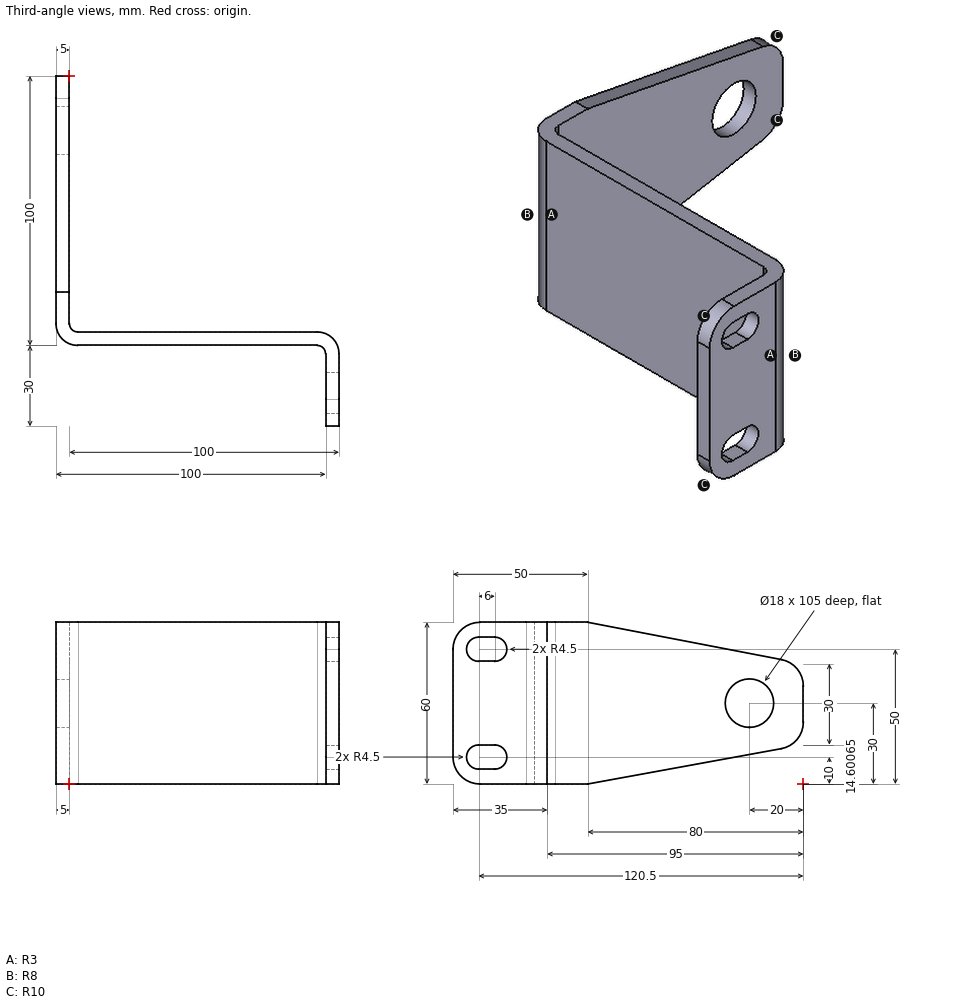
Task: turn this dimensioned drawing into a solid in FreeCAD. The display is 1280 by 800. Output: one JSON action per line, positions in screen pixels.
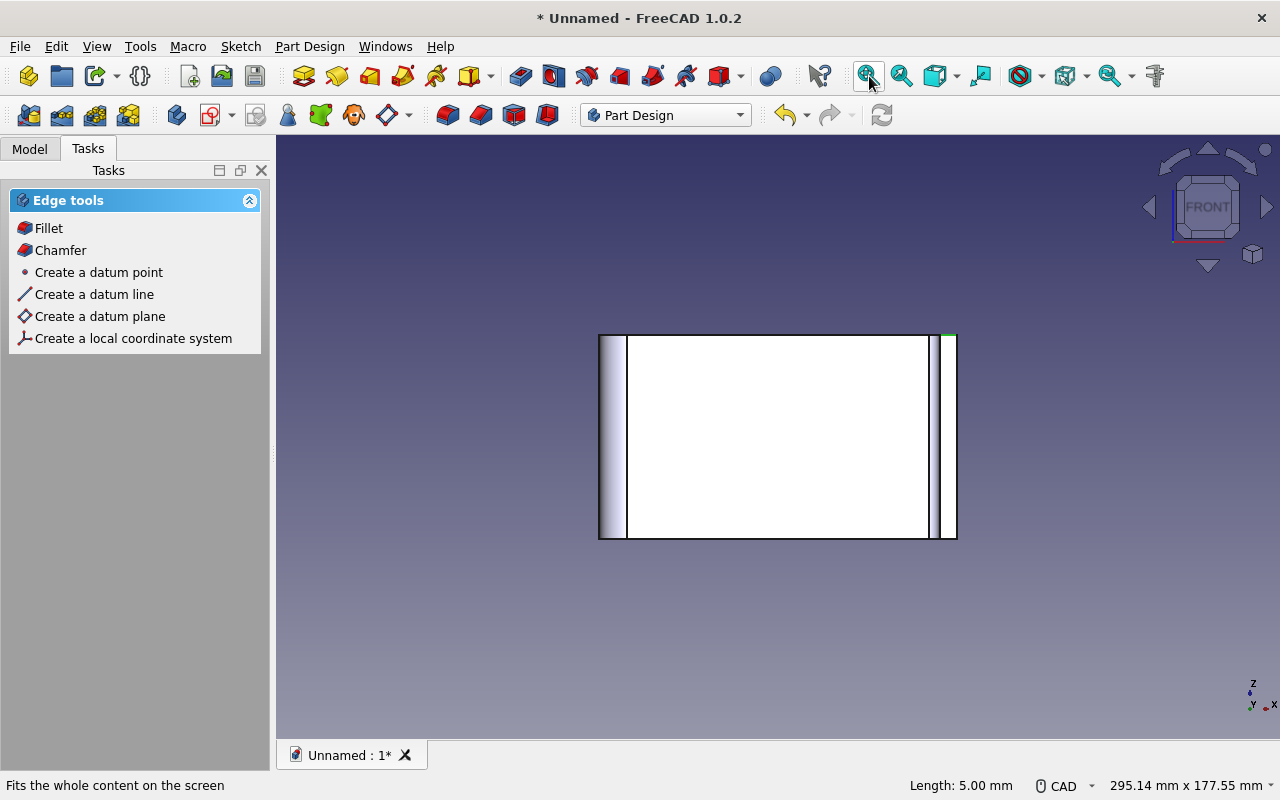
{"action": "left_click", "coordinate": [869, 76]}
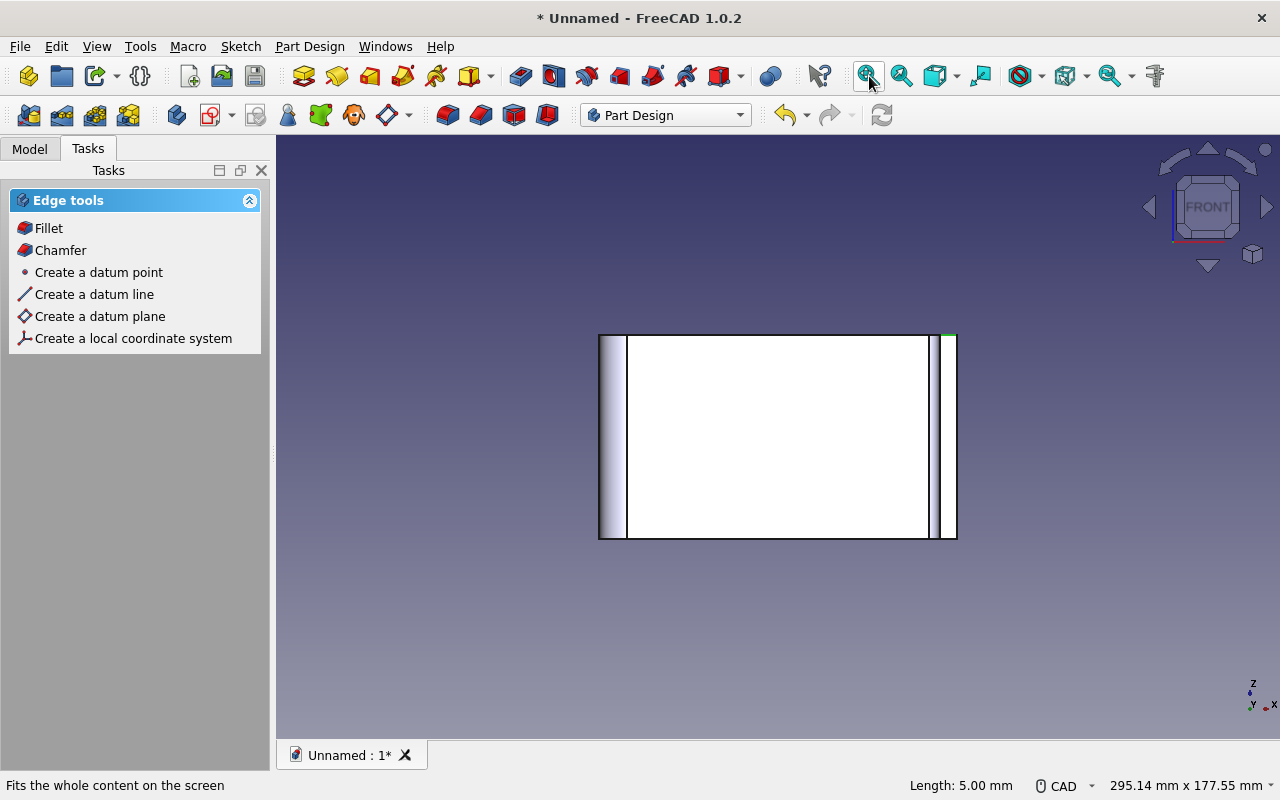
{"action": "left_click", "coordinate": [948, 538], "text": "ctrl"}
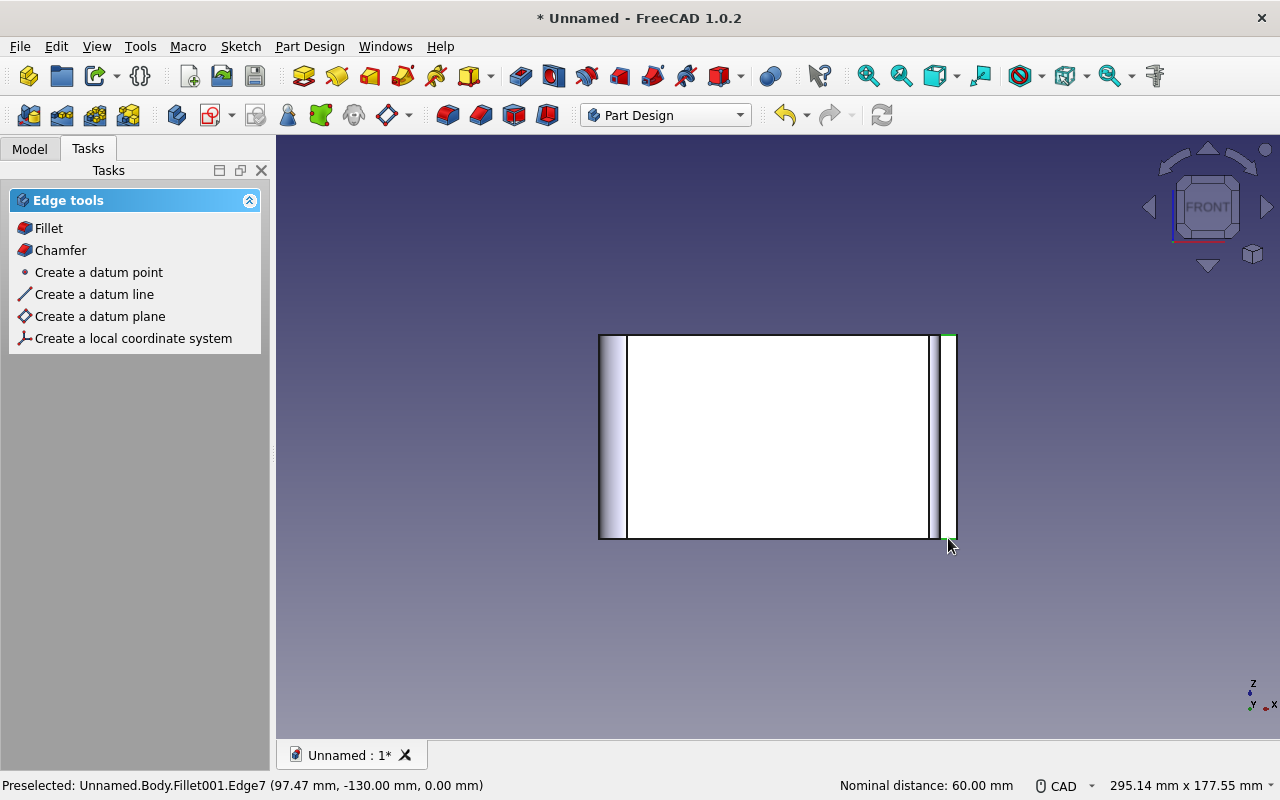
{"action": "scroll", "coordinate": [608, 386], "scroll_direction": "up", "scroll_amount": 5}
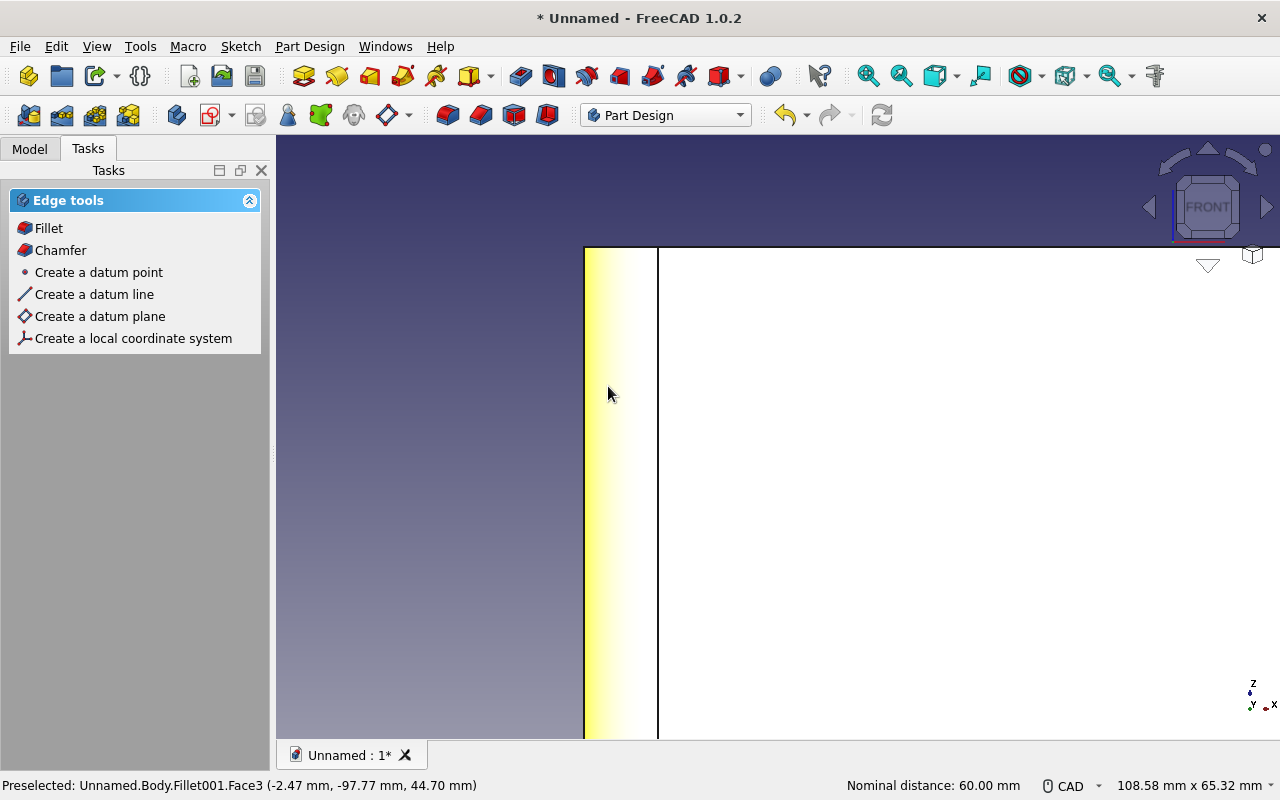
{"action": "left_click", "coordinate": [869, 76]}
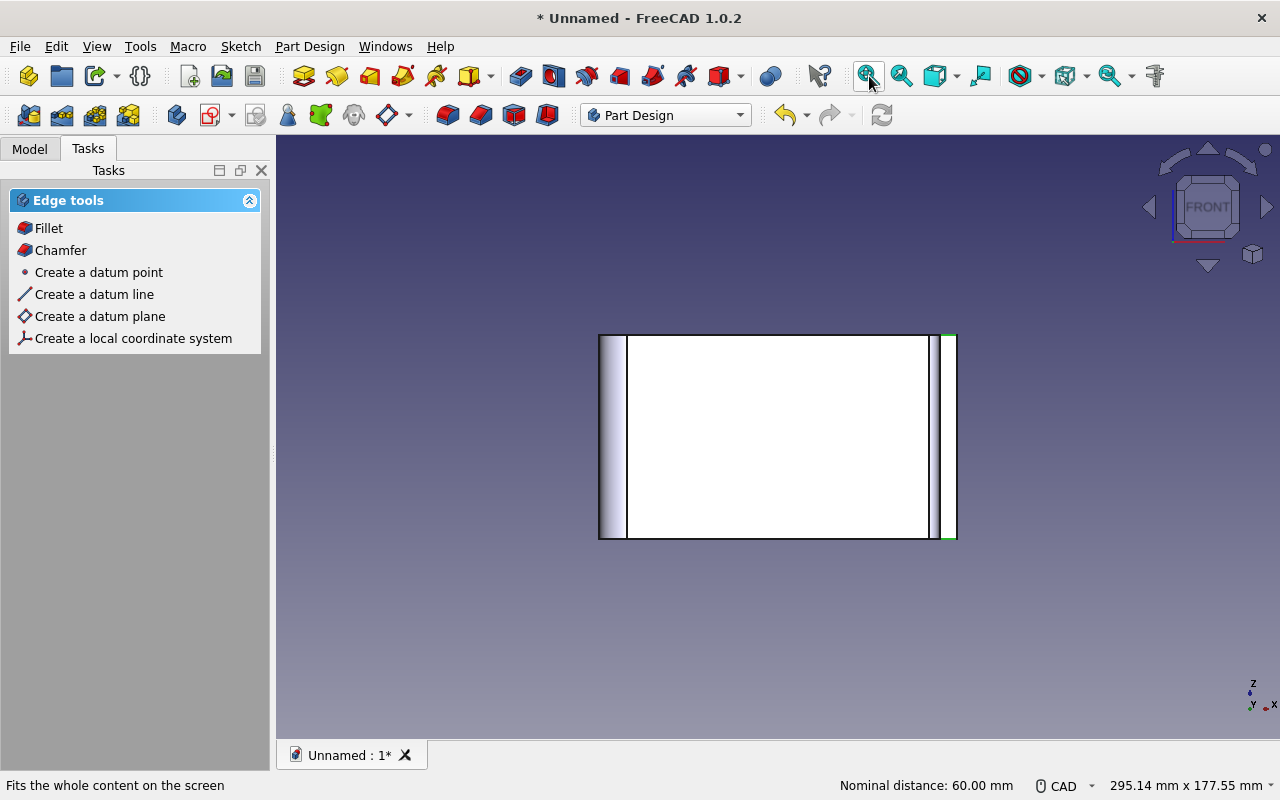
{"action": "key", "text": "3"}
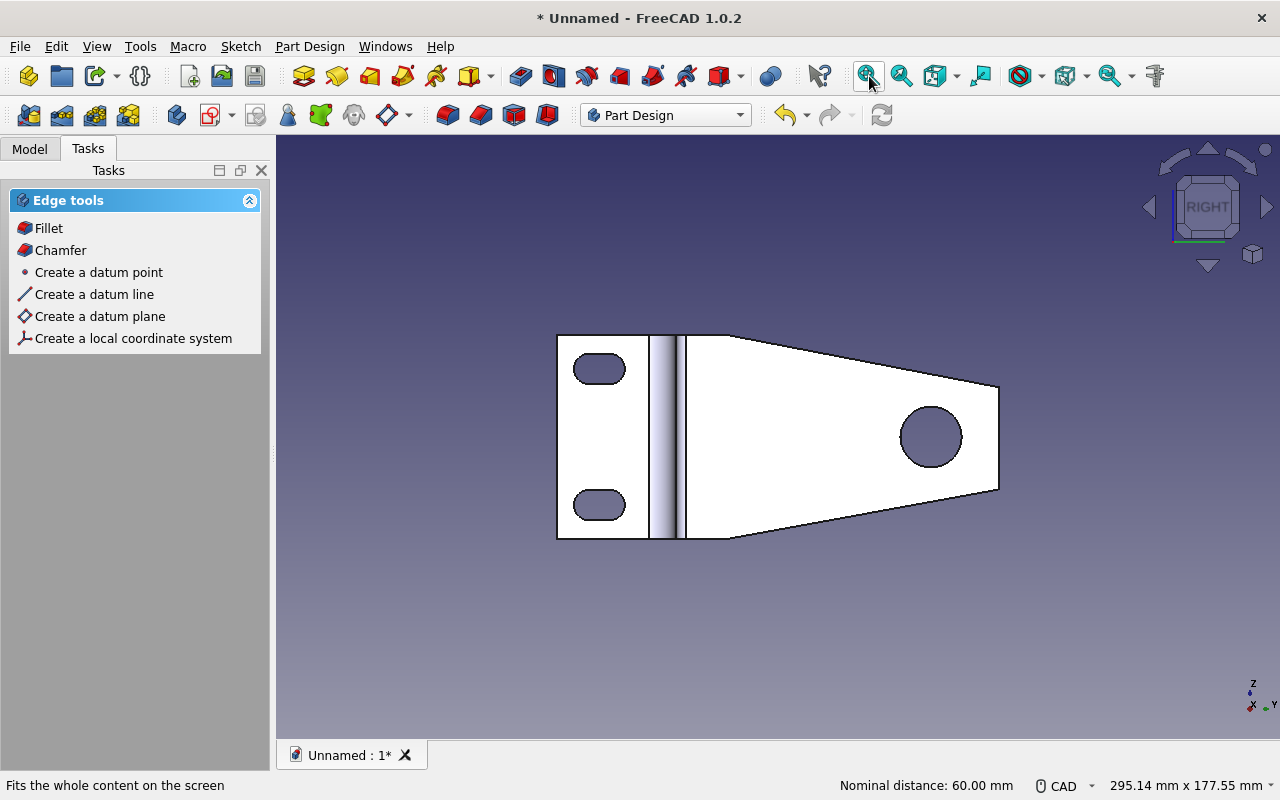
{"action": "left_click", "coordinate": [869, 76]}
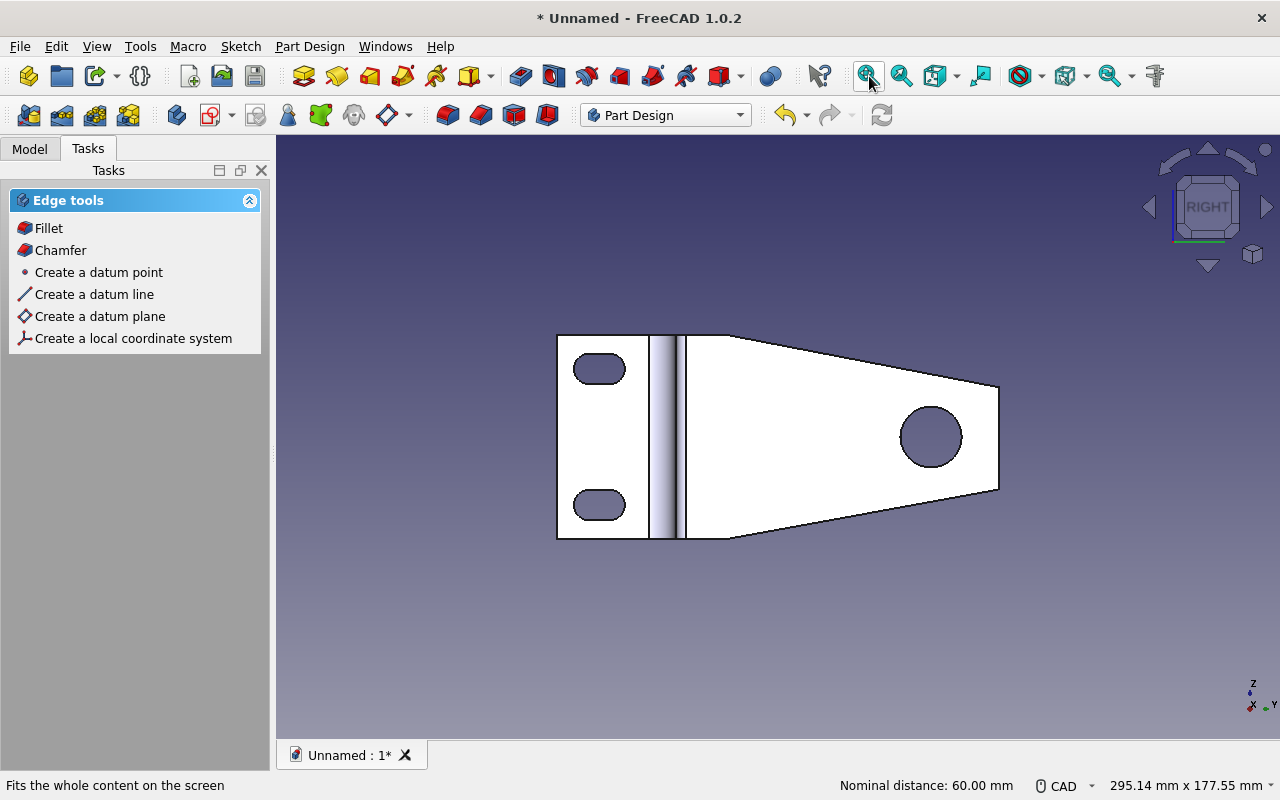
{"action": "scroll", "coordinate": [999, 386], "scroll_direction": "up", "scroll_amount": 5}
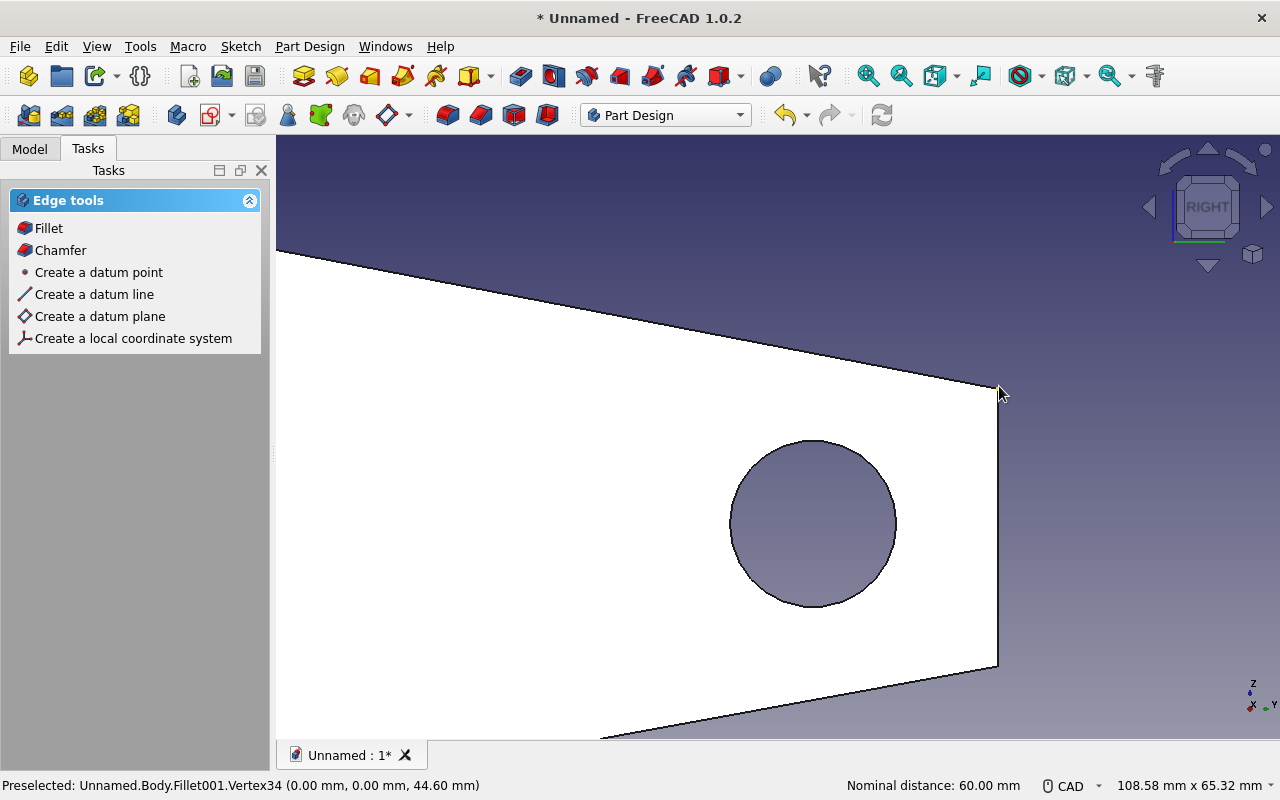
{"action": "left_click", "coordinate": [869, 76]}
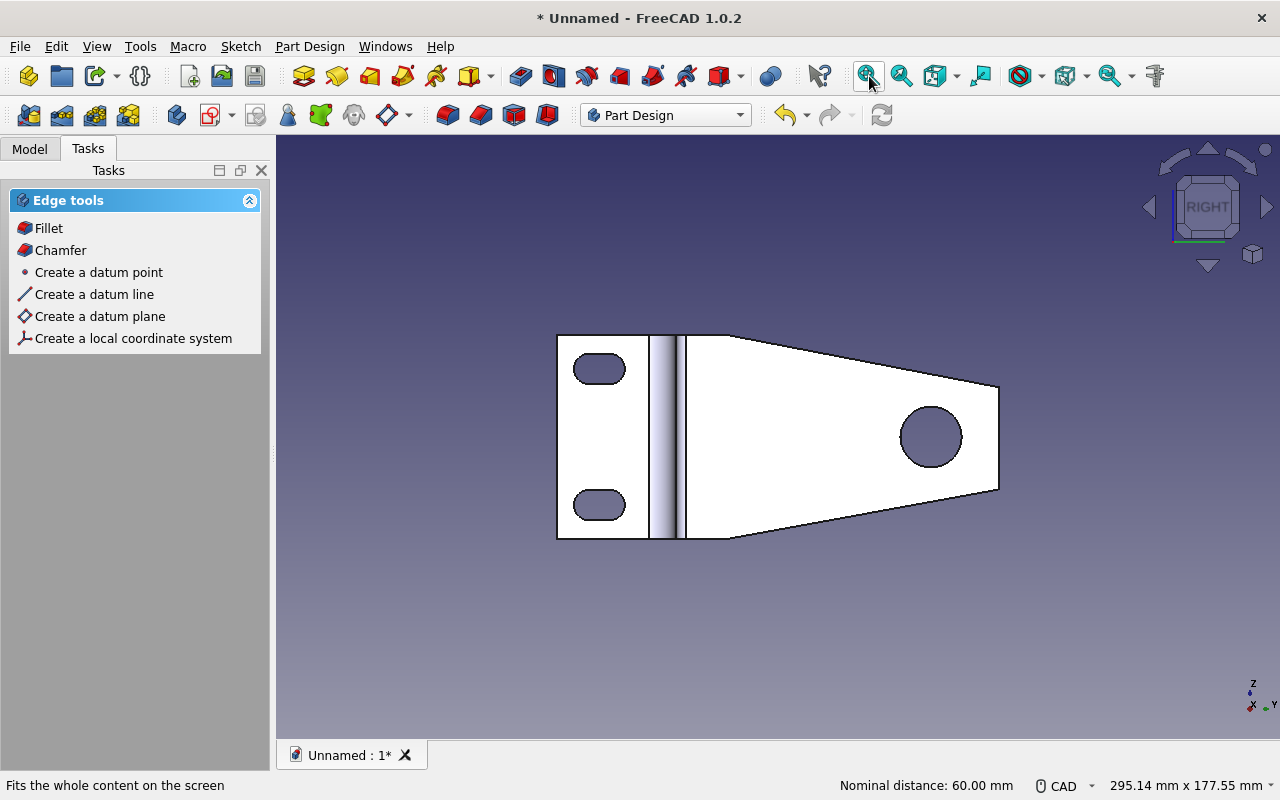
{"action": "key", "text": "5"}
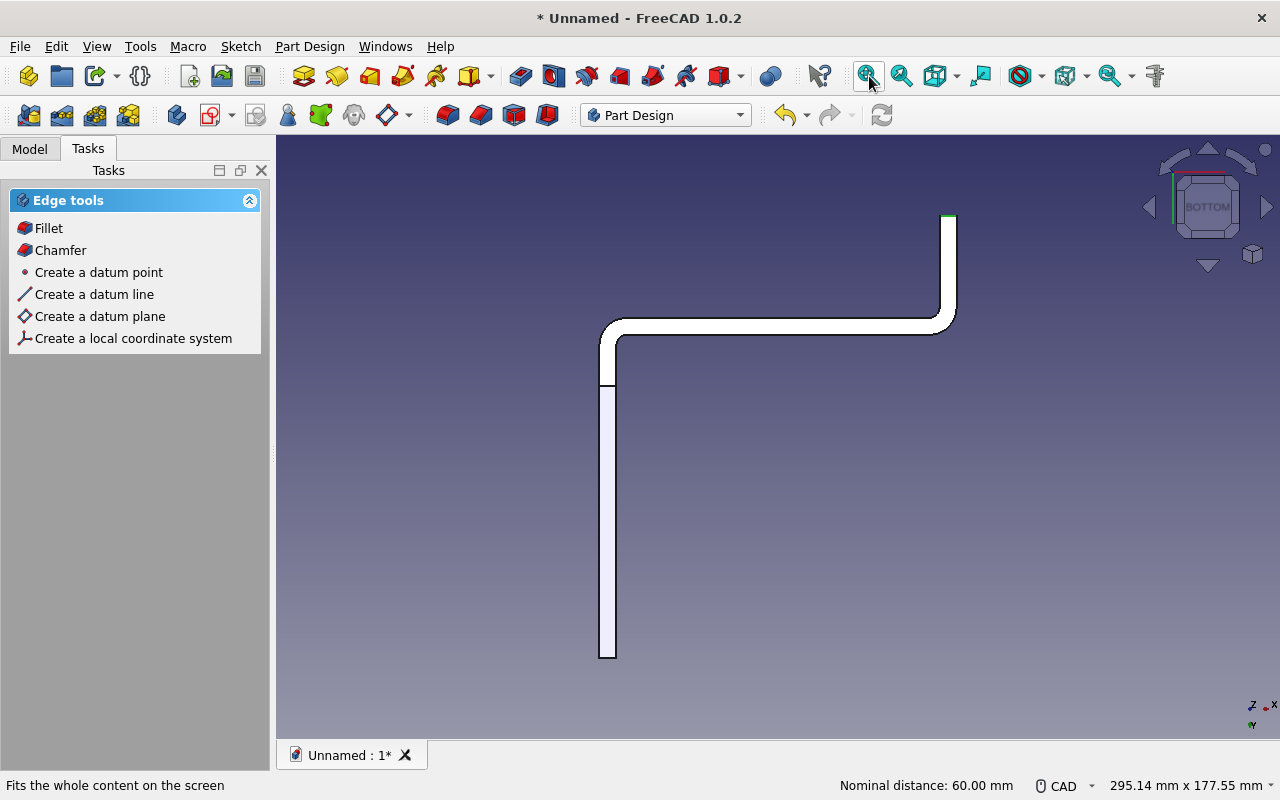
{"action": "scroll", "coordinate": [608, 657], "scroll_direction": "up", "scroll_amount": 5}